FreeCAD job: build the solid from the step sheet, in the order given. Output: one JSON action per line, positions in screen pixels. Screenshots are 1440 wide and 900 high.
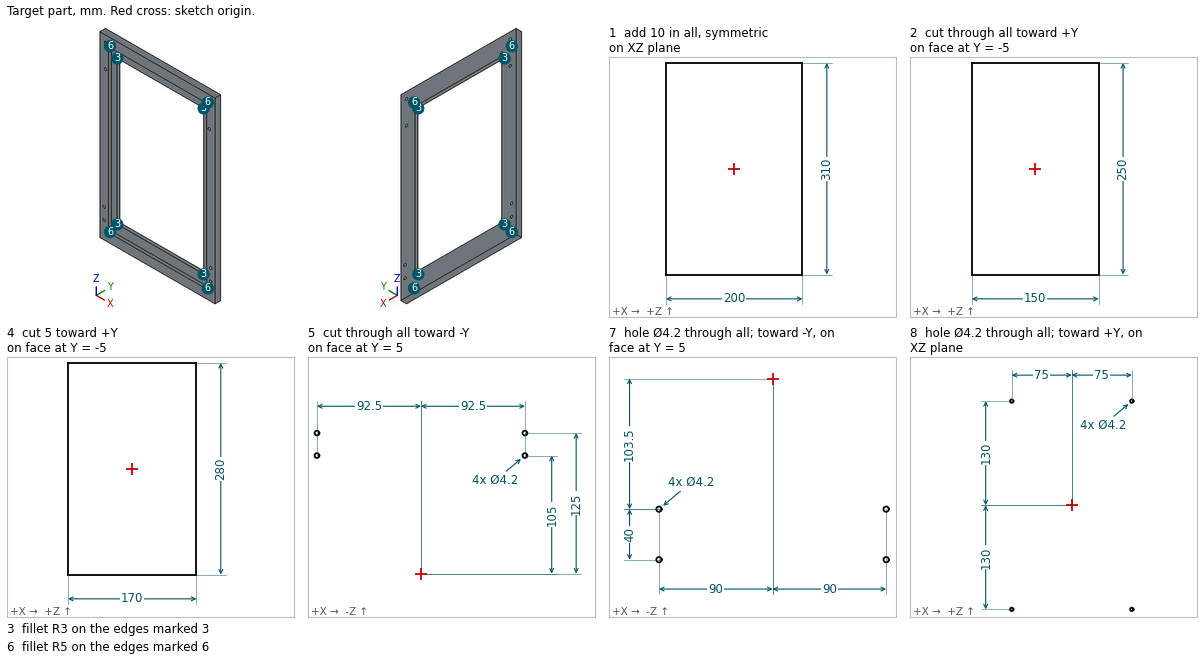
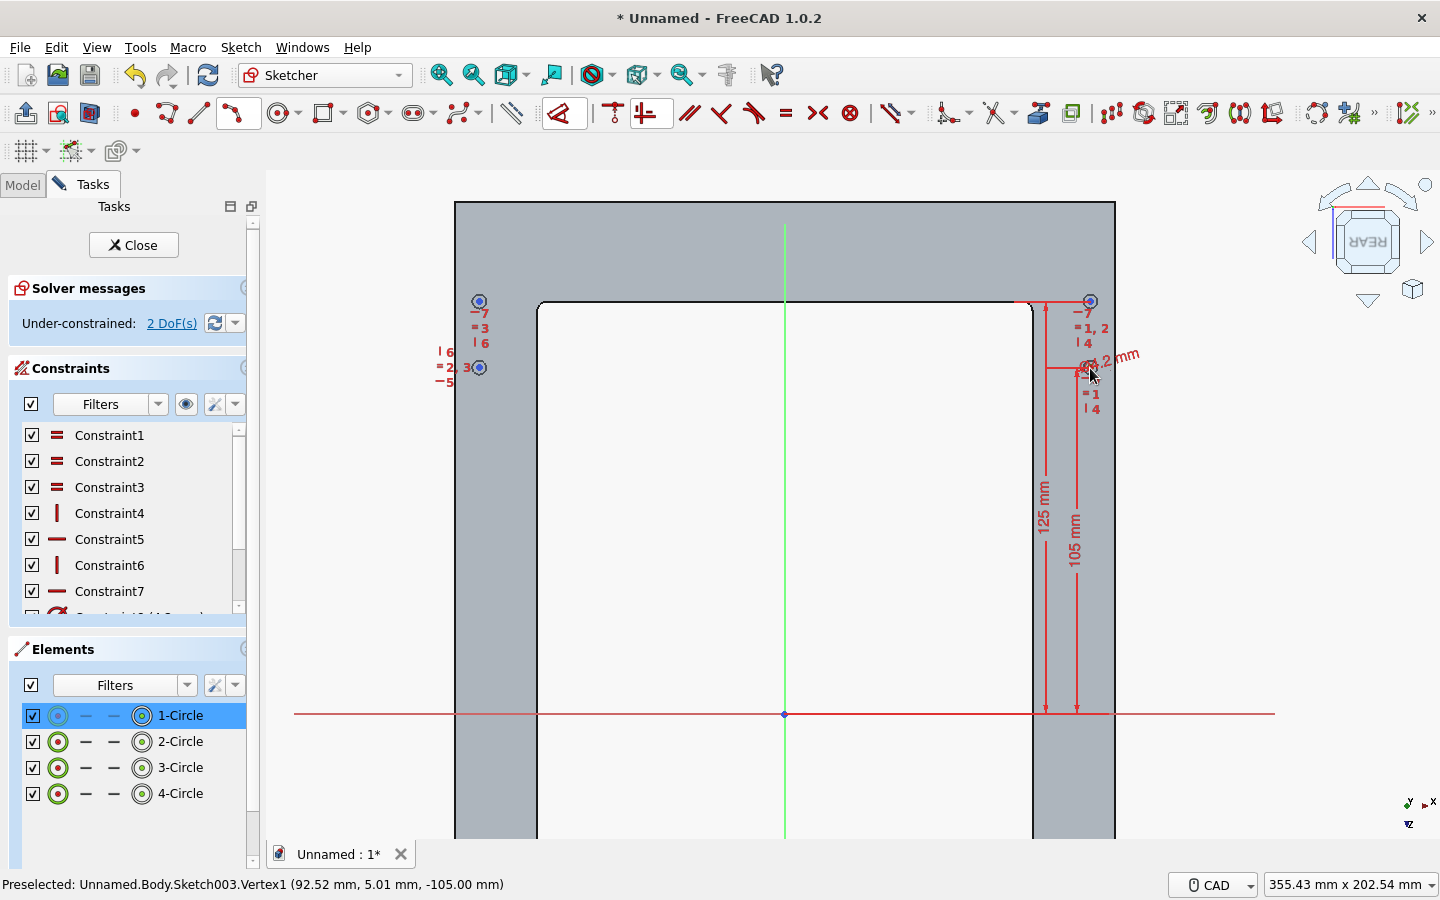
{"action": "key", "text": "l"}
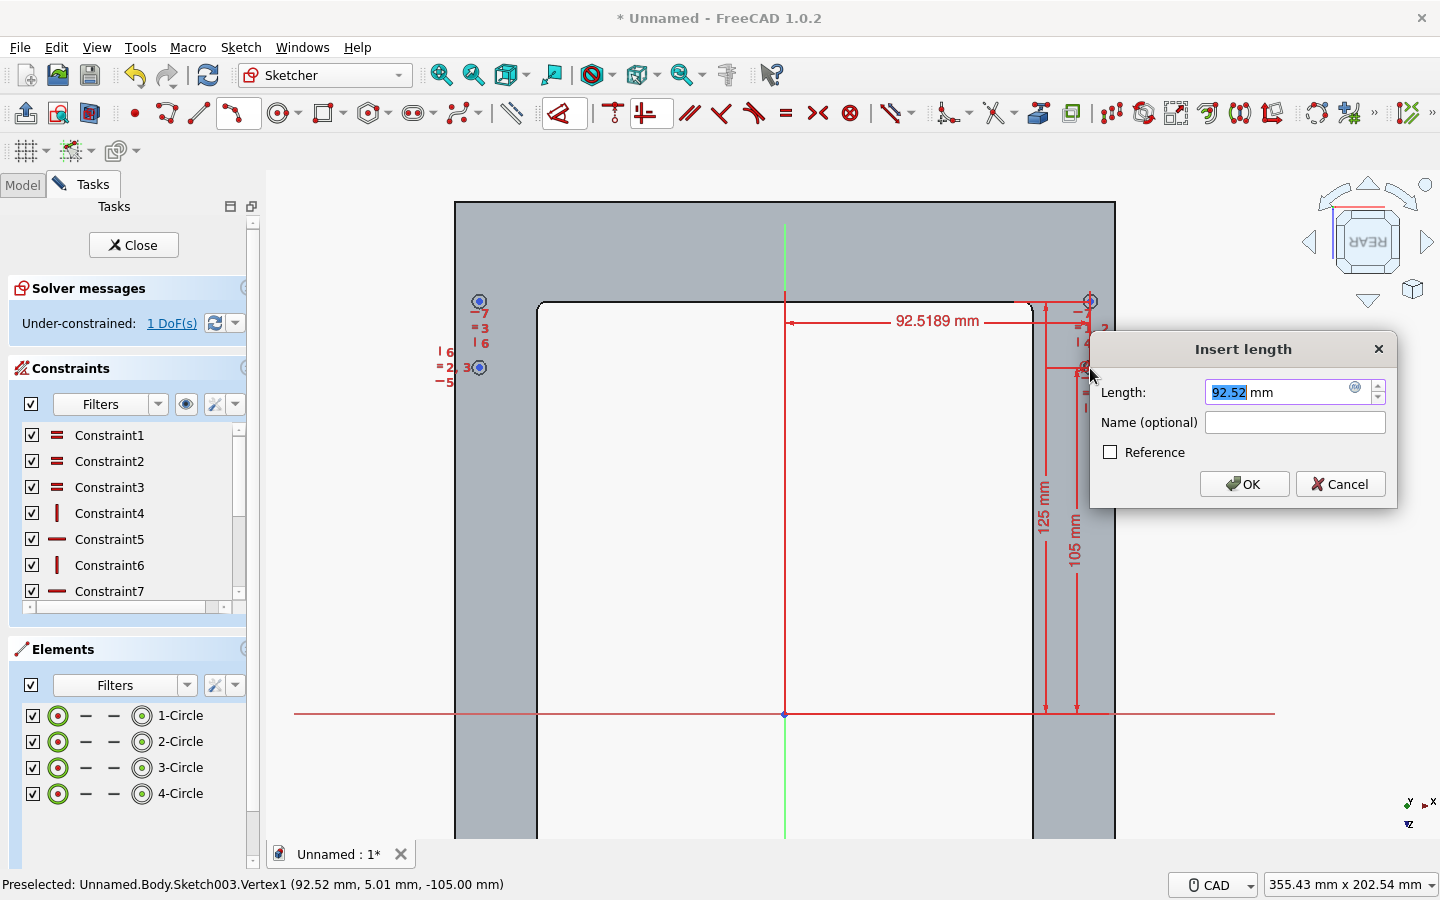
{"action": "type", "text": "92.5"}
{"action": "key", "text": "Return"}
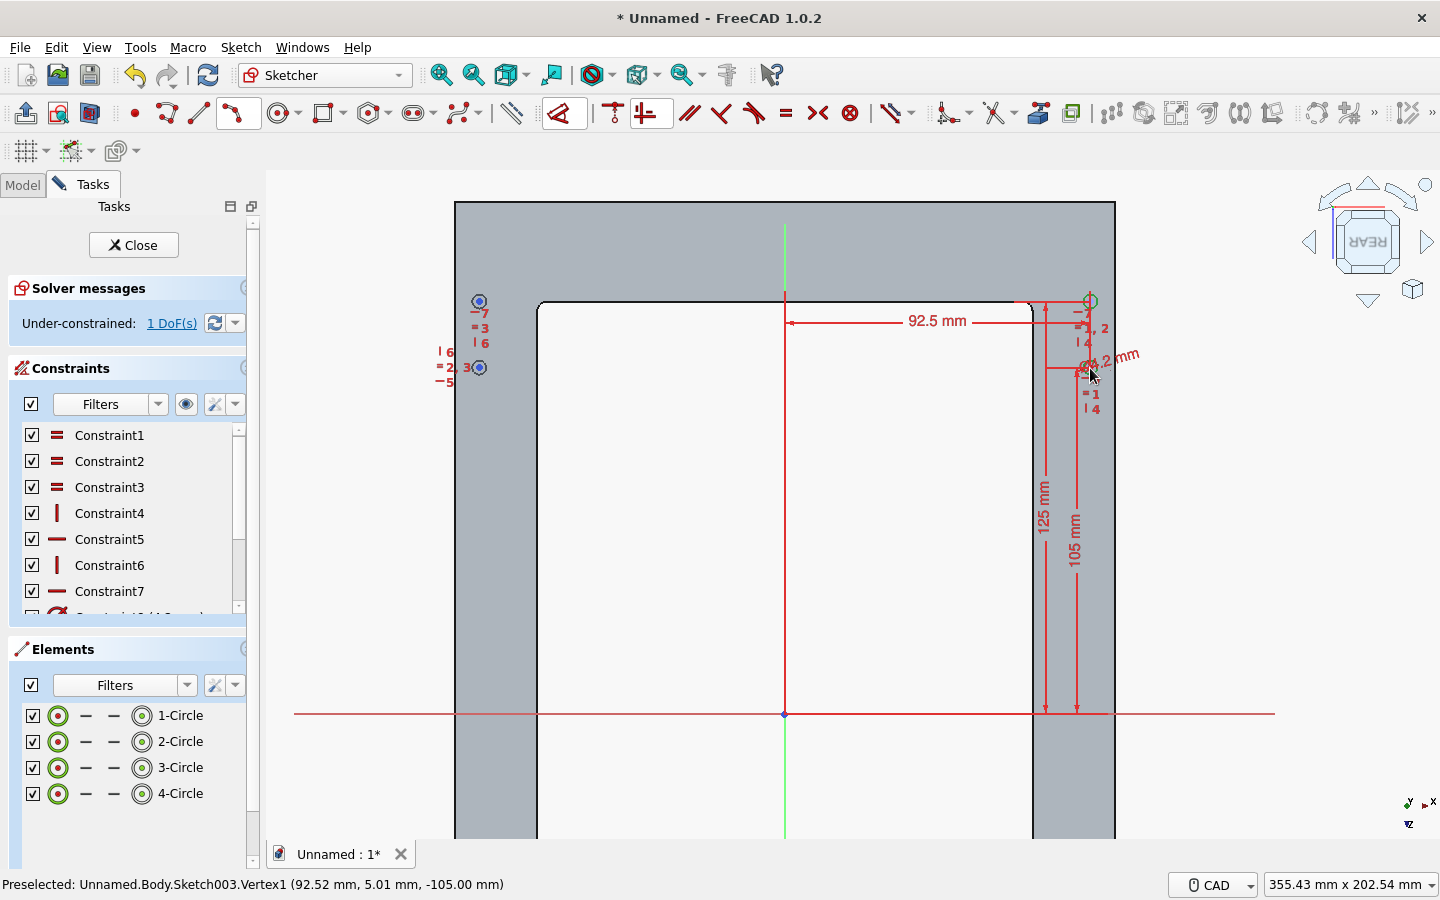
{"action": "left_click", "coordinate": [479, 368]}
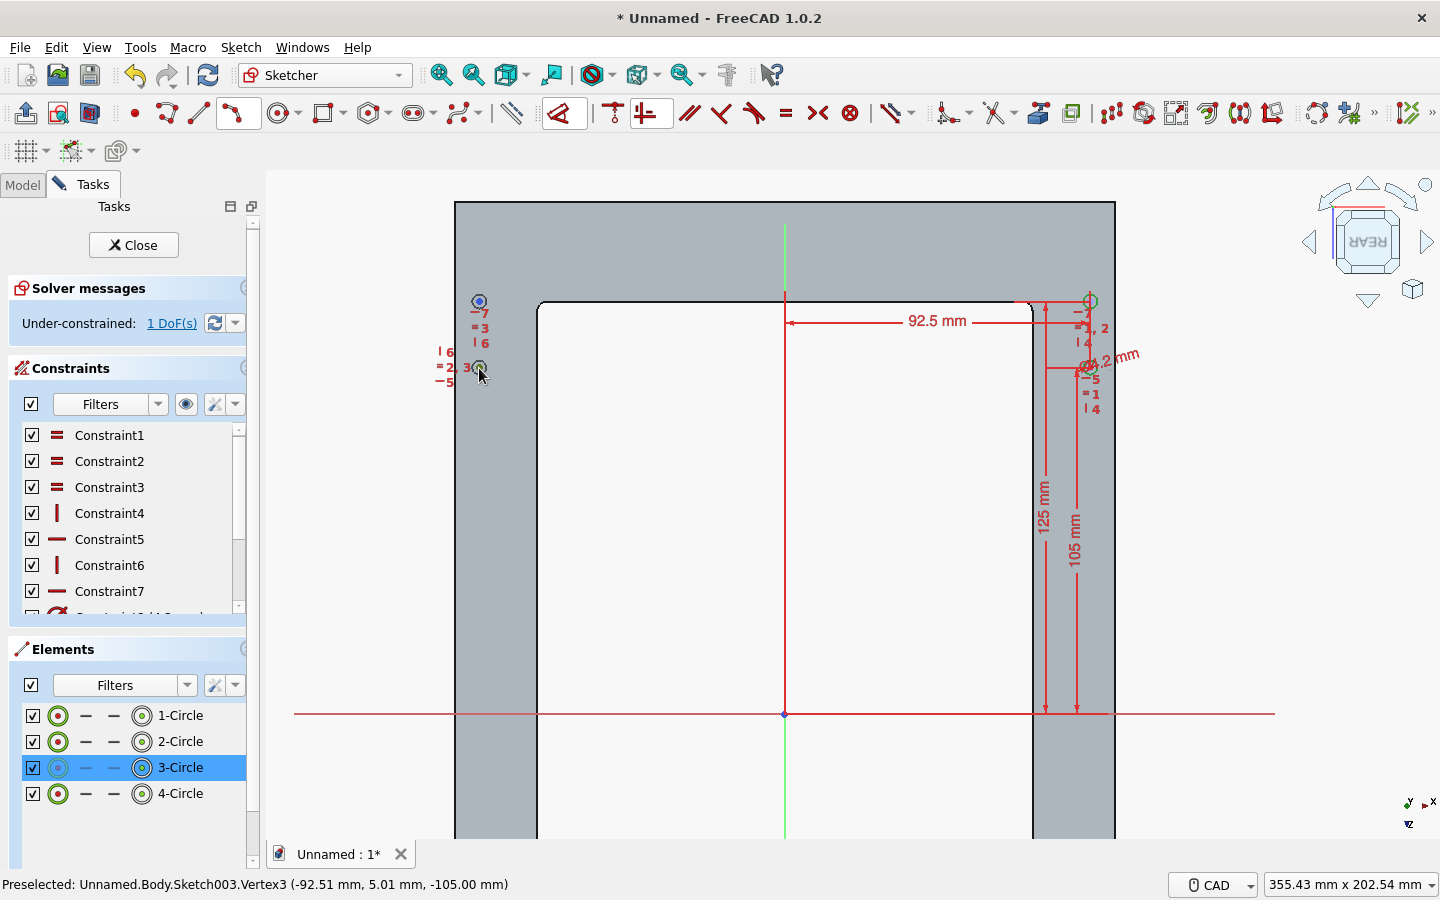
{"action": "key", "text": "l"}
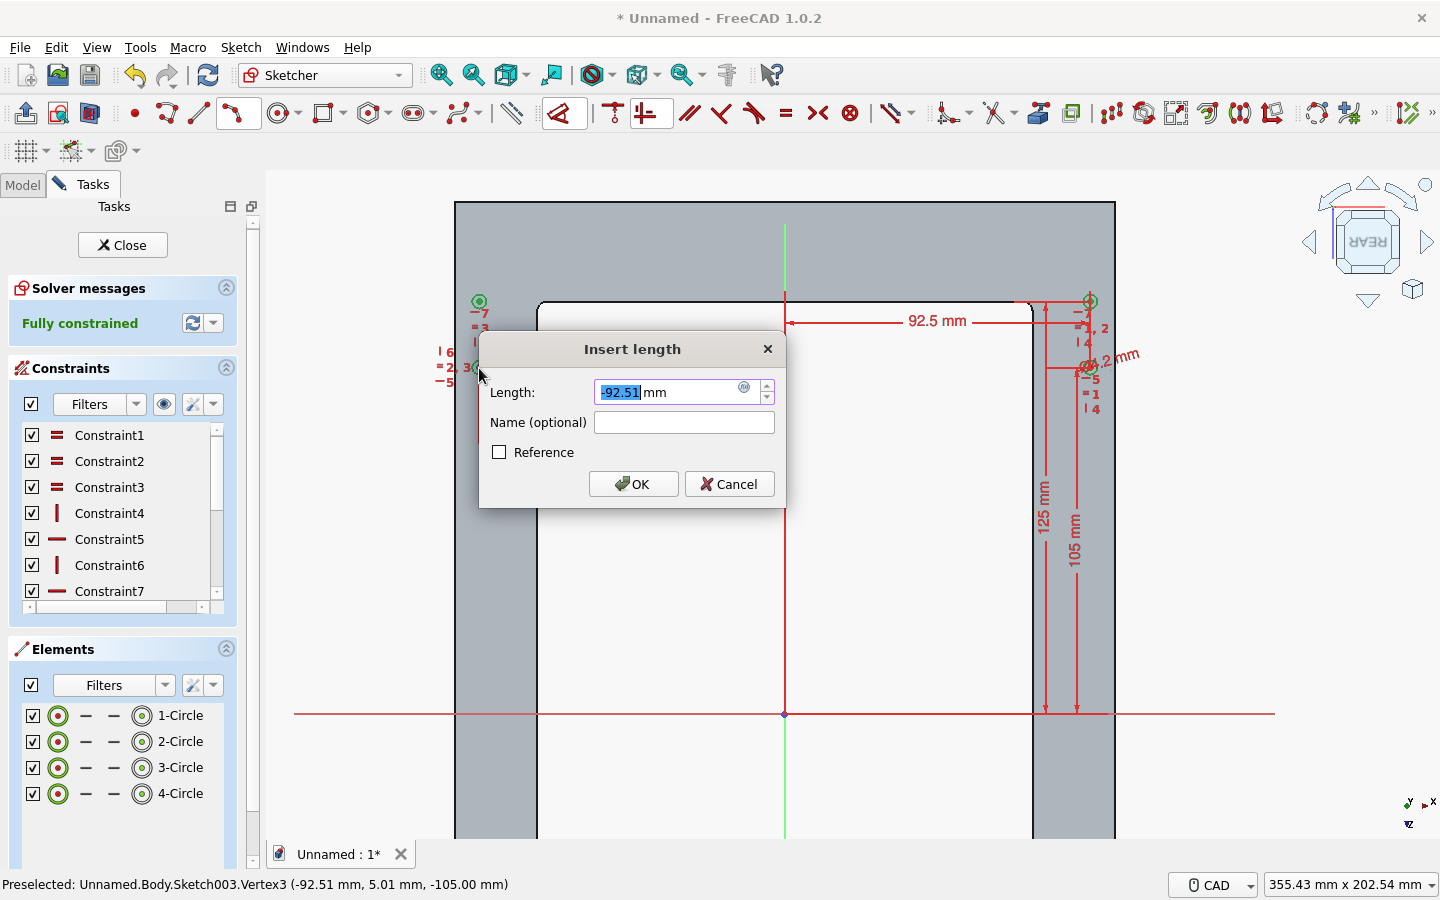
{"action": "type", "text": "-92.5"}
{"action": "key", "text": "Return"}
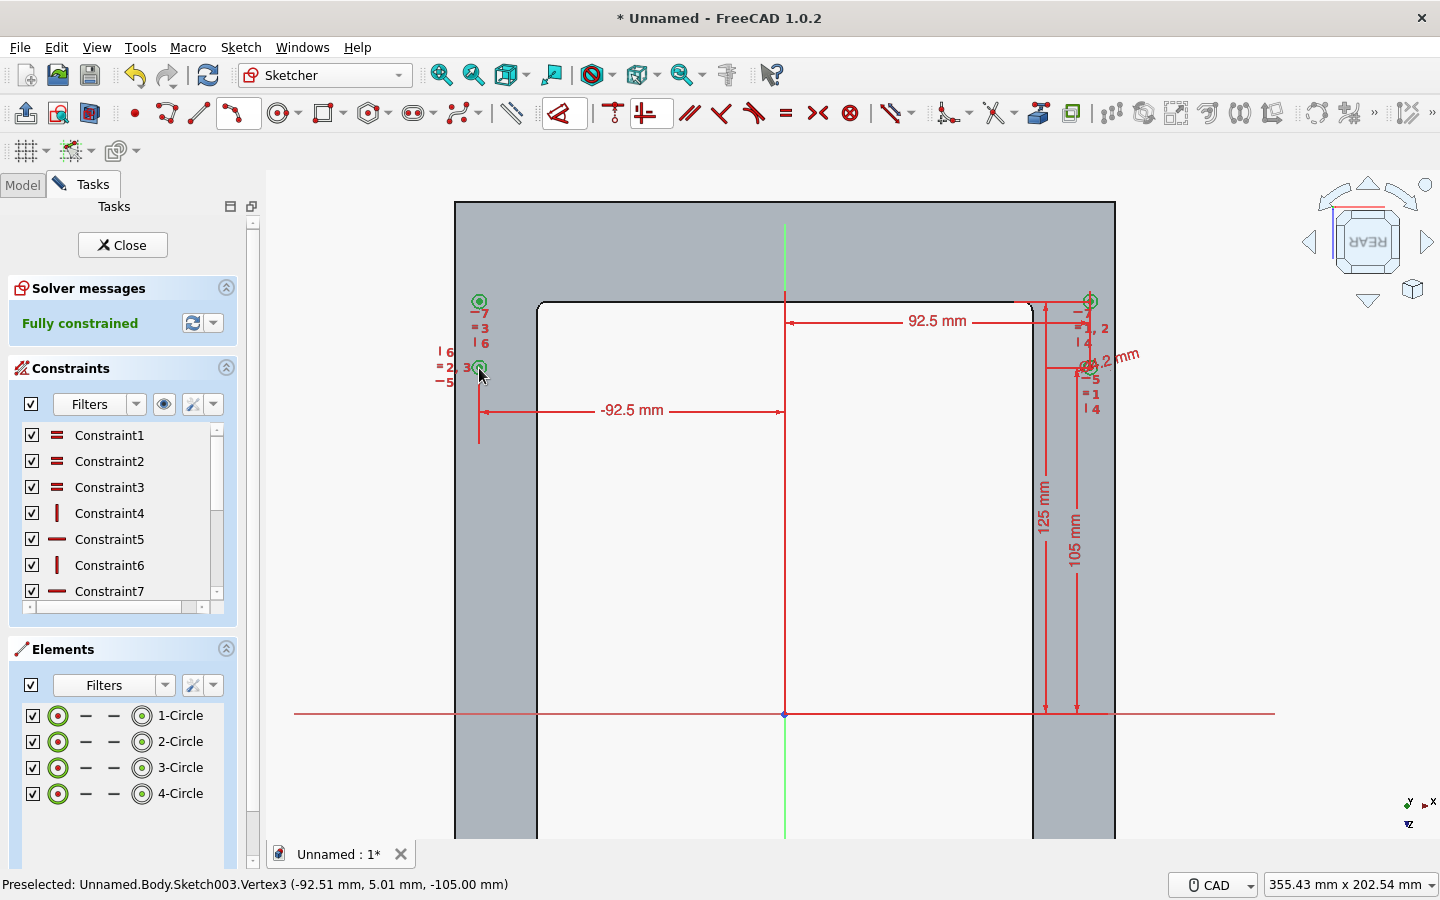
{"action": "left_click", "coordinate": [123, 245]}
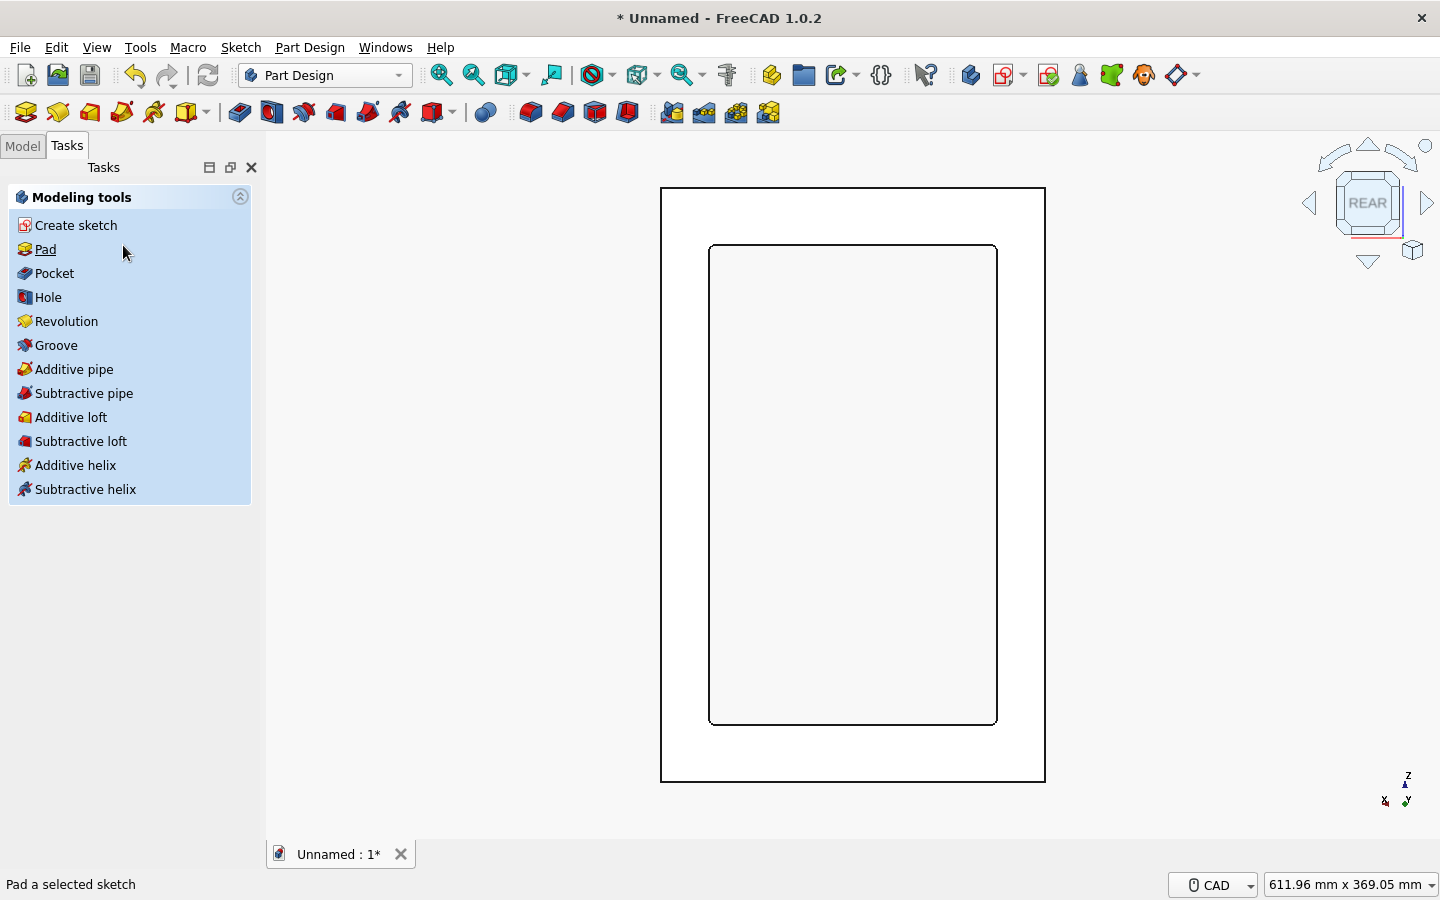
{"action": "left_click", "coordinate": [240, 112]}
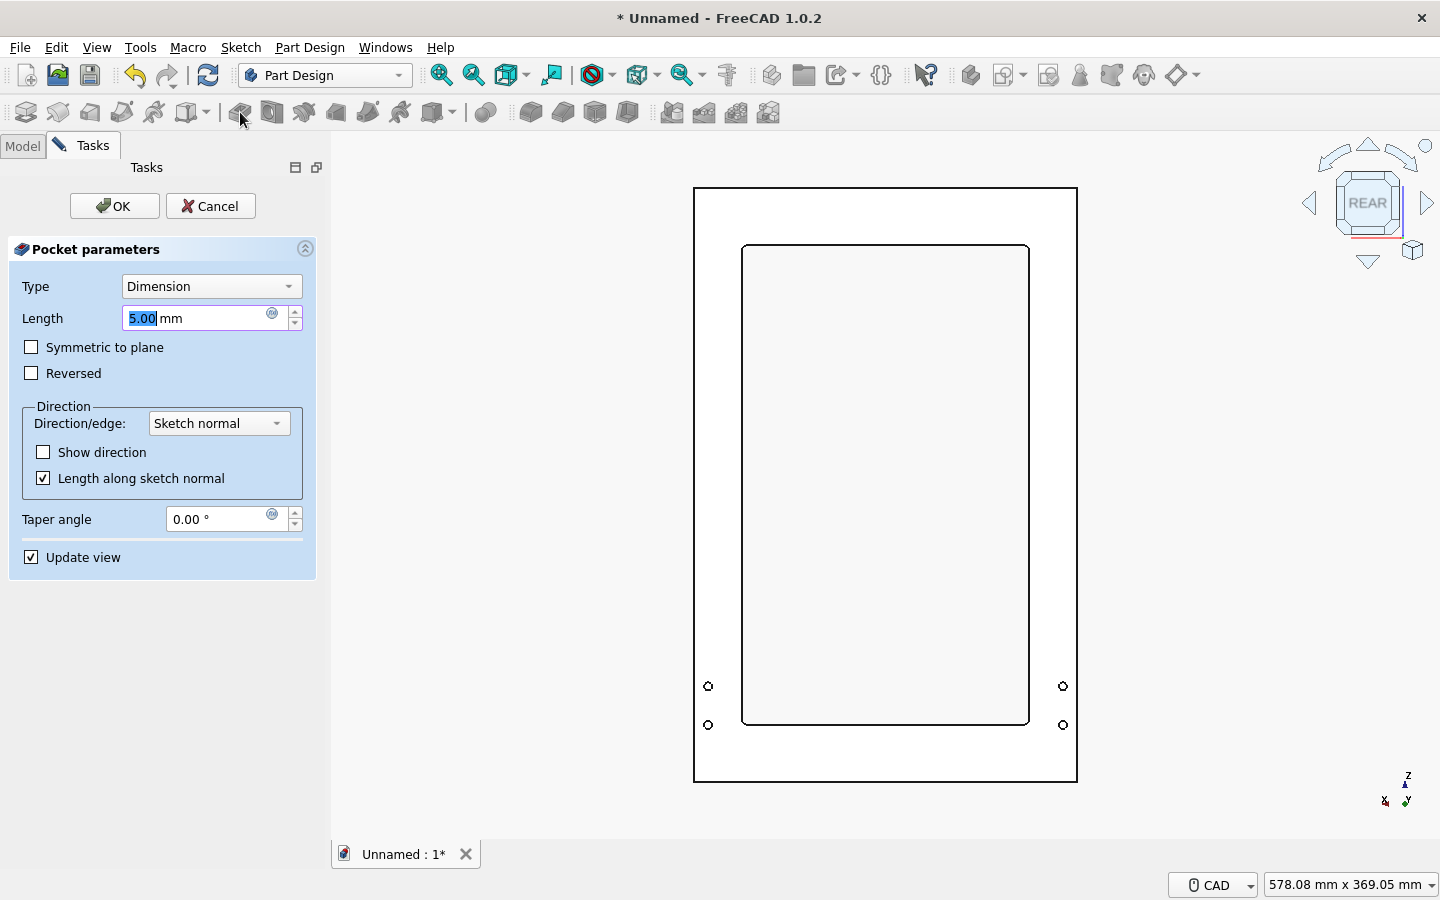
{"action": "left_click", "coordinate": [212, 286]}